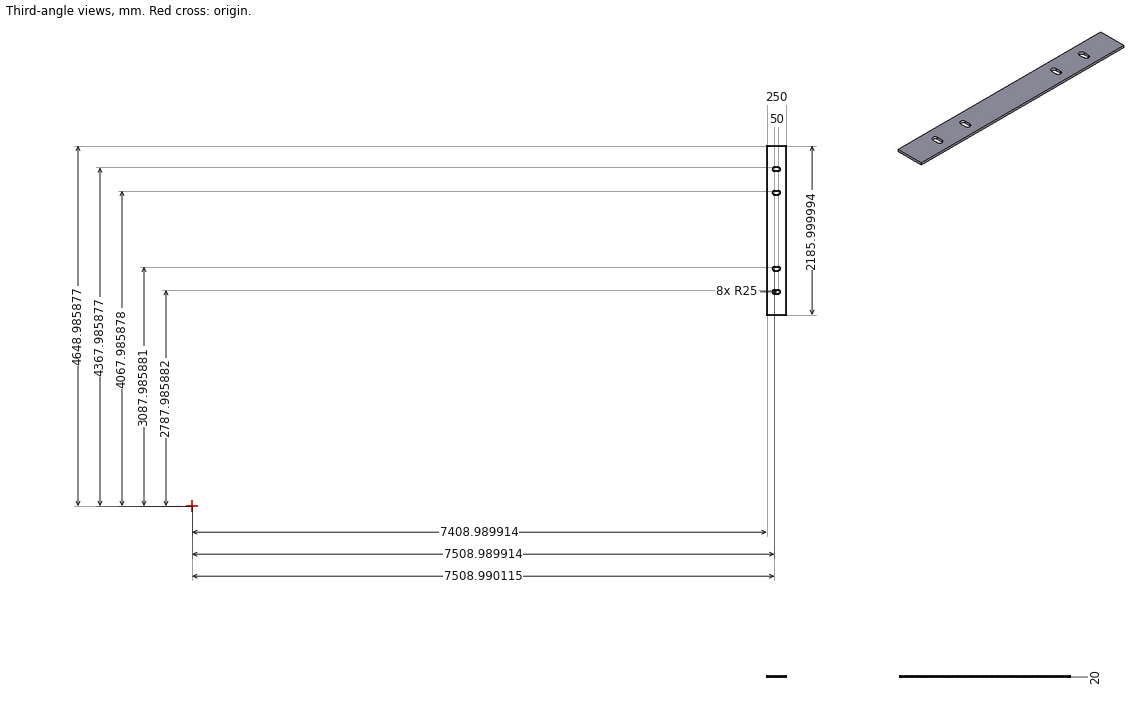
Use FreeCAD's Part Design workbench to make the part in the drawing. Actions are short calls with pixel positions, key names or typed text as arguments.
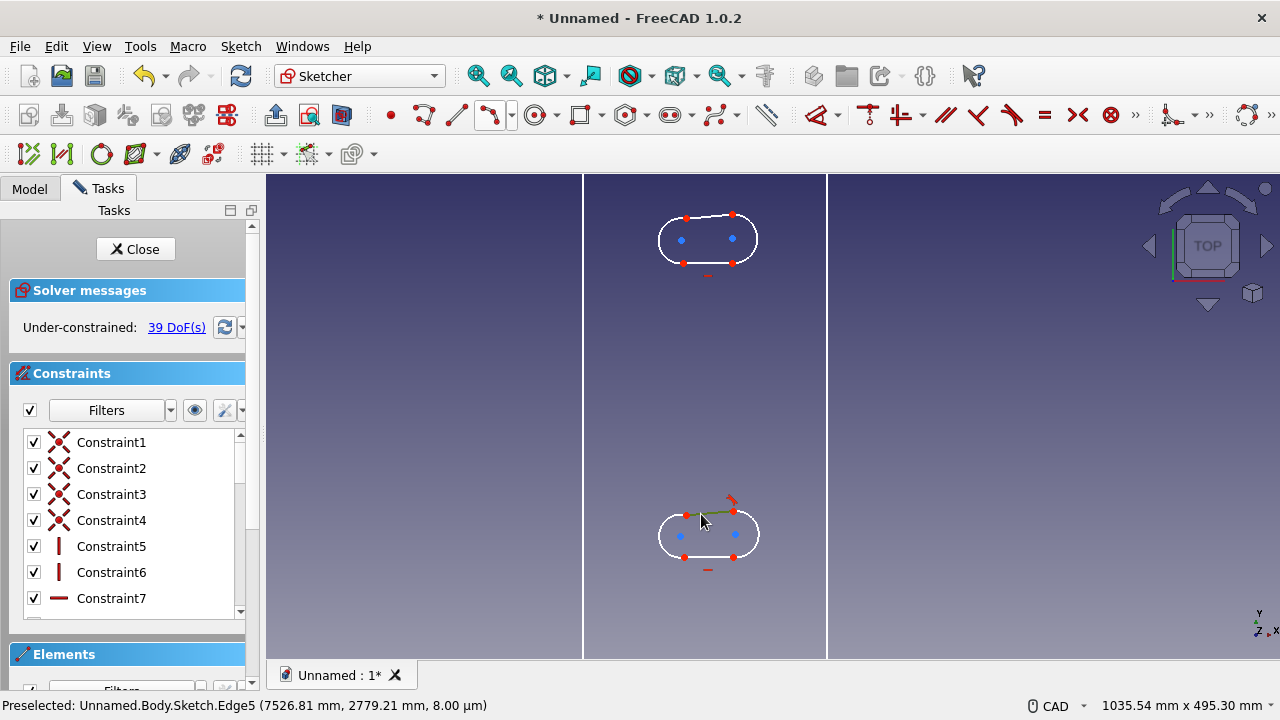
click(665, 521)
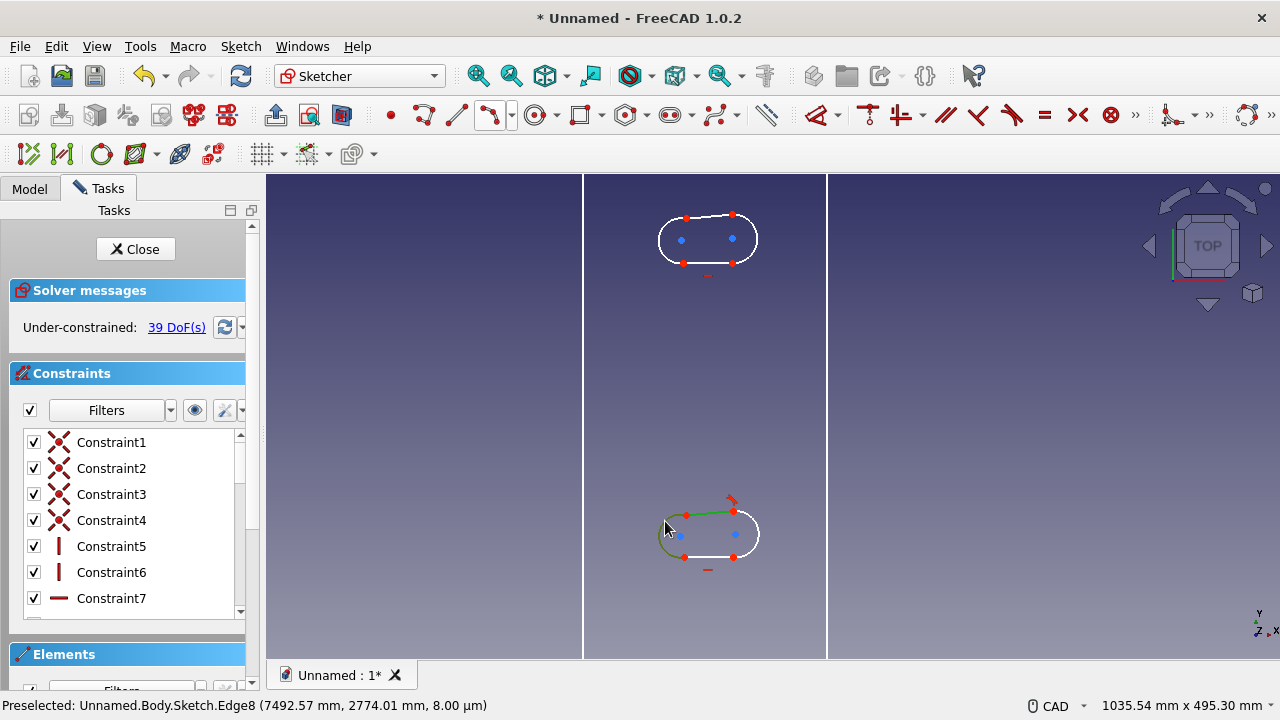
click(1012, 116)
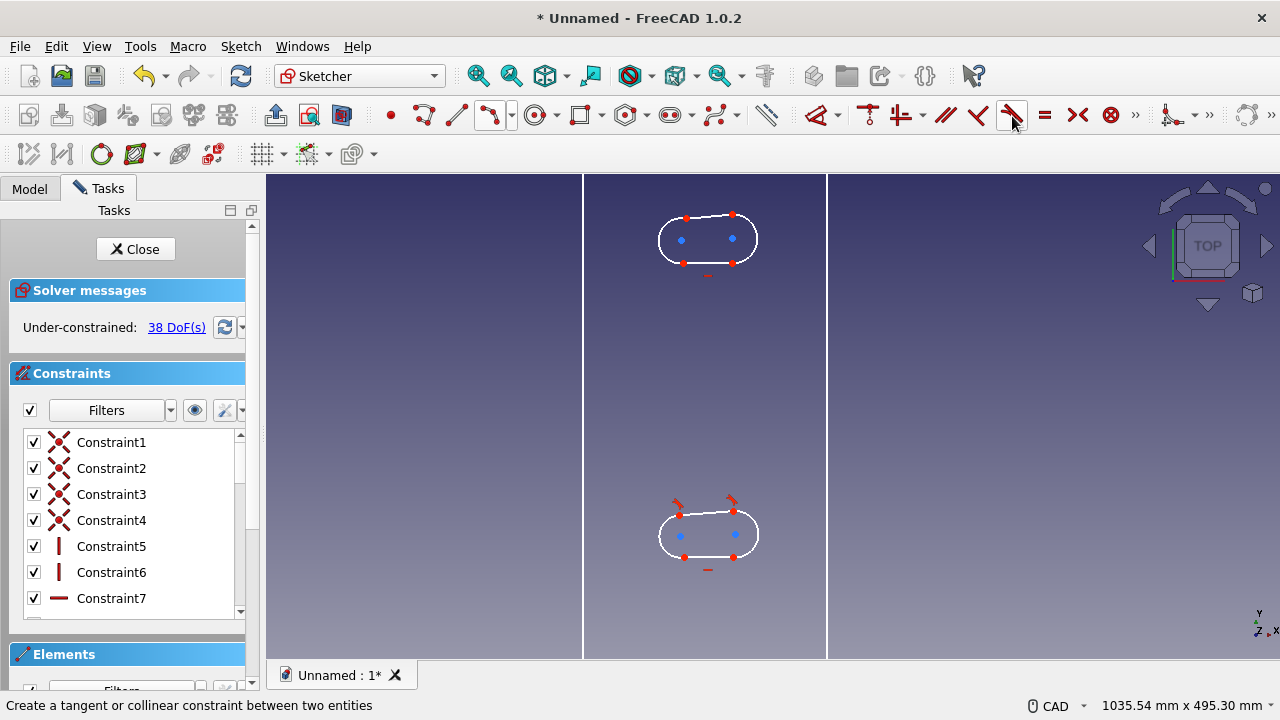
click(719, 557)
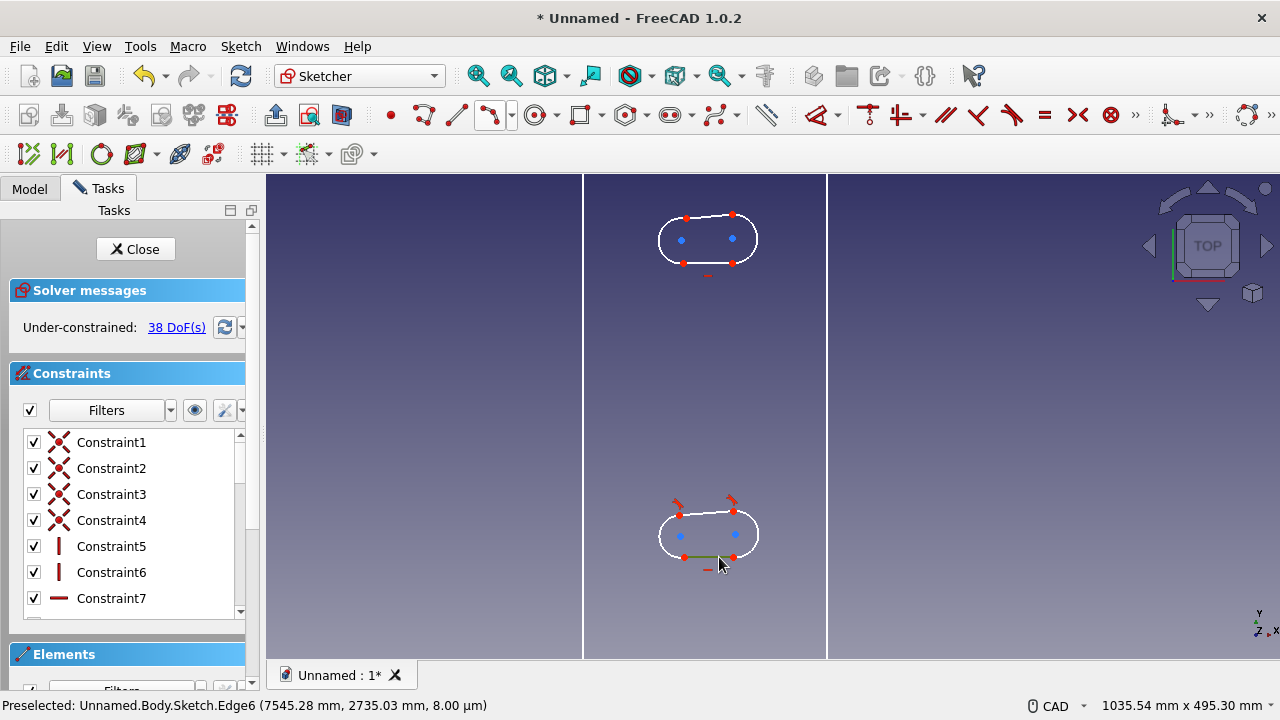
click(754, 548)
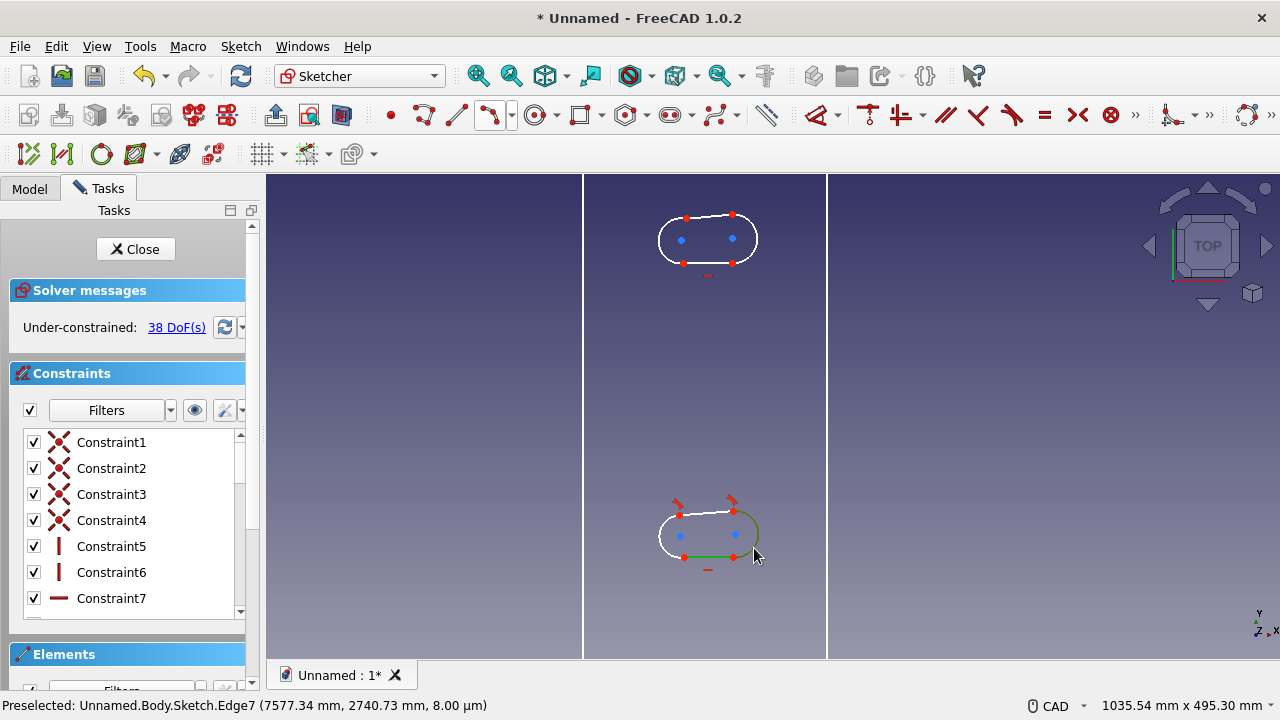
key(t)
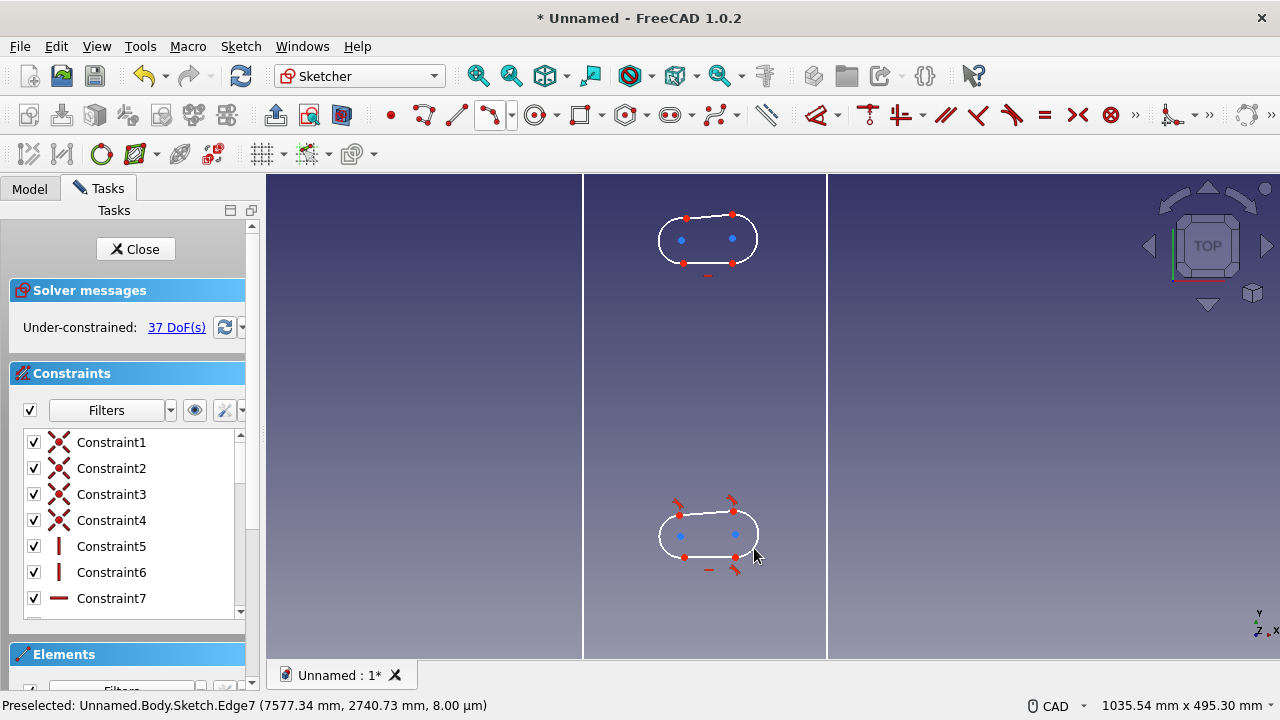
click(720, 557)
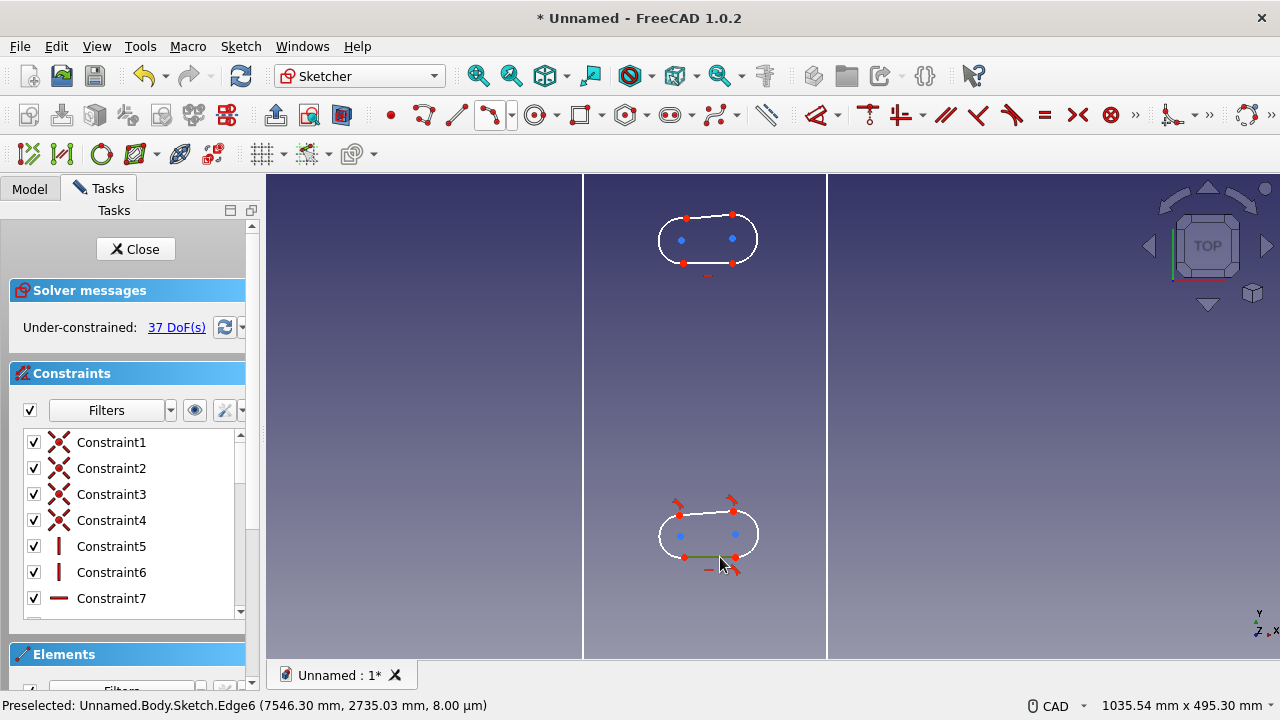
click(662, 526)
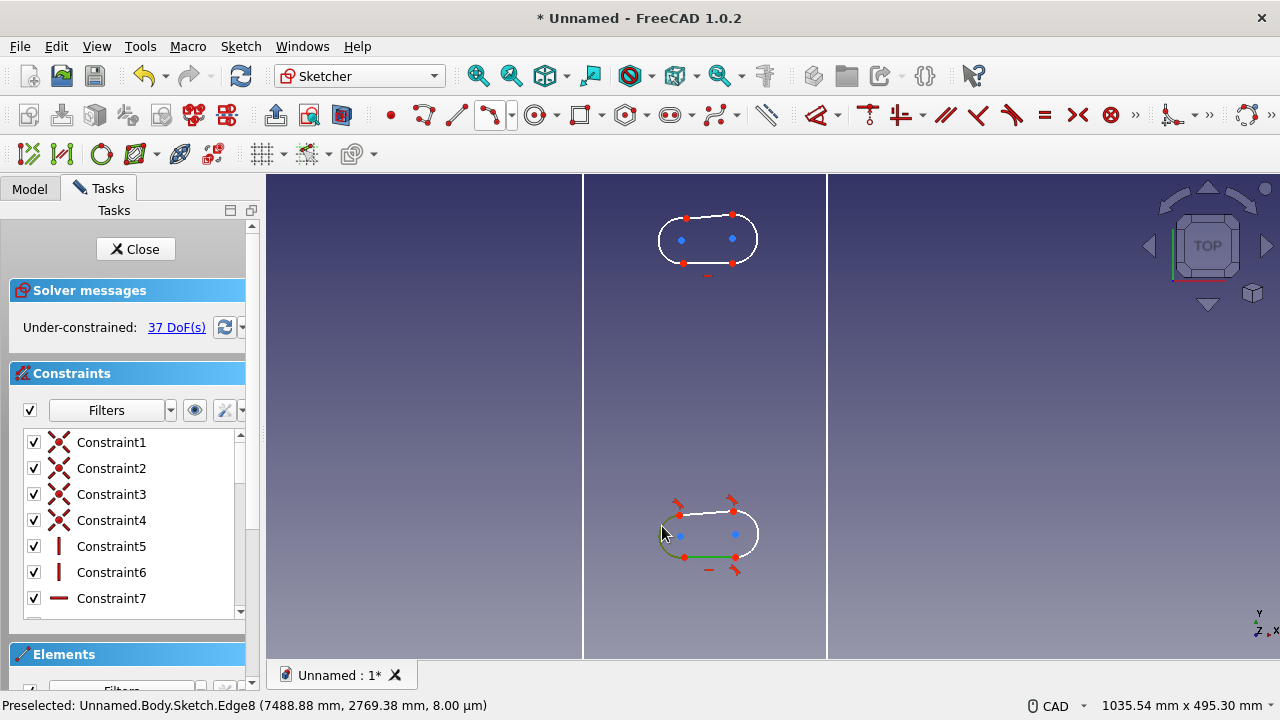
click(1012, 116)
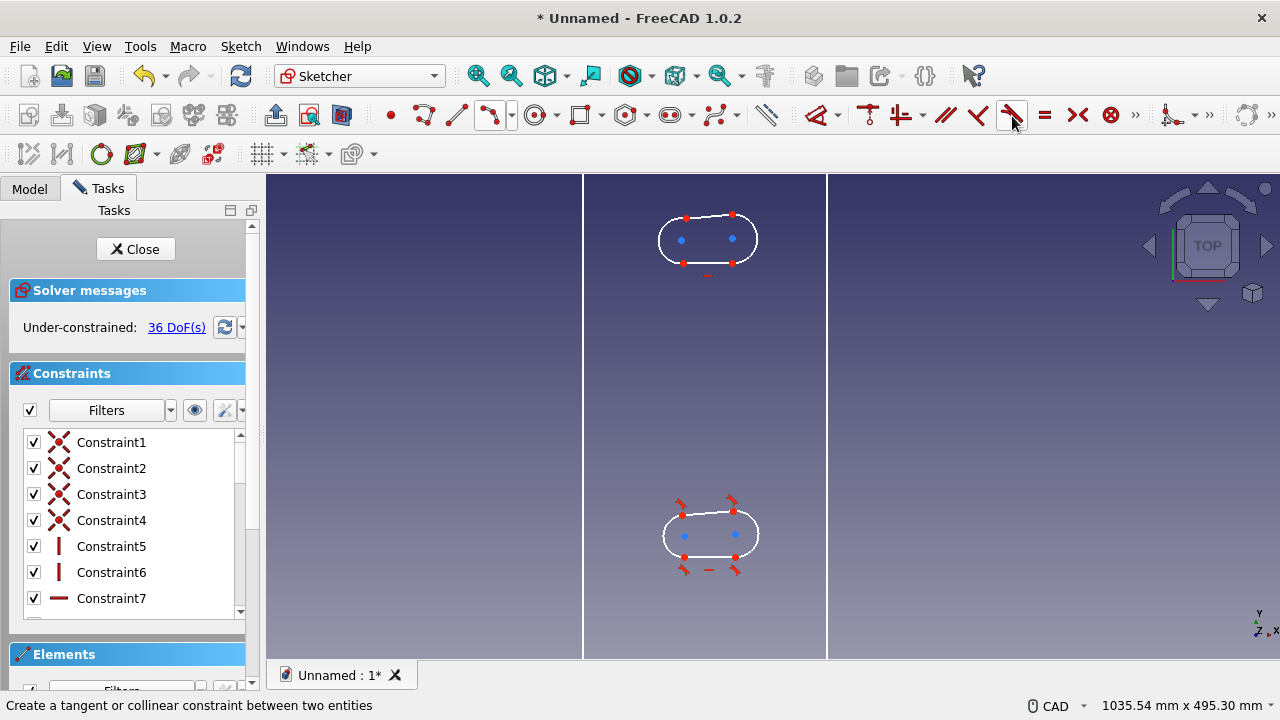
click(700, 218)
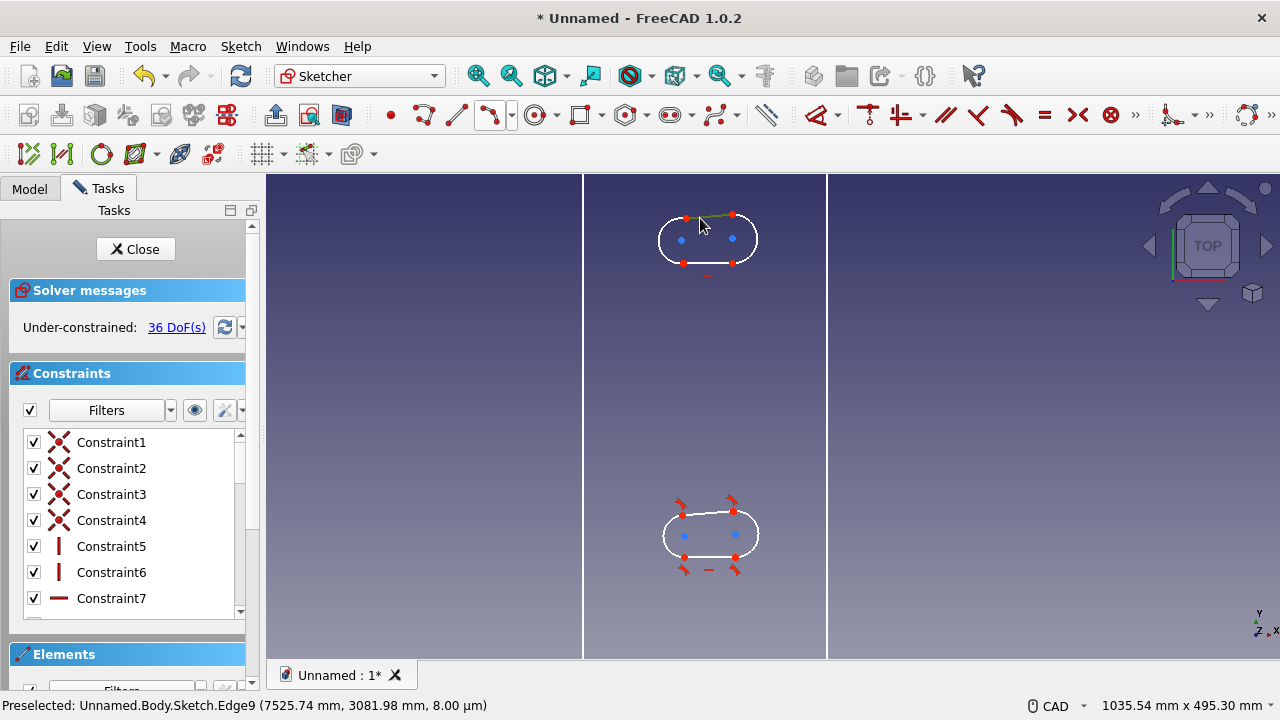
click(753, 253)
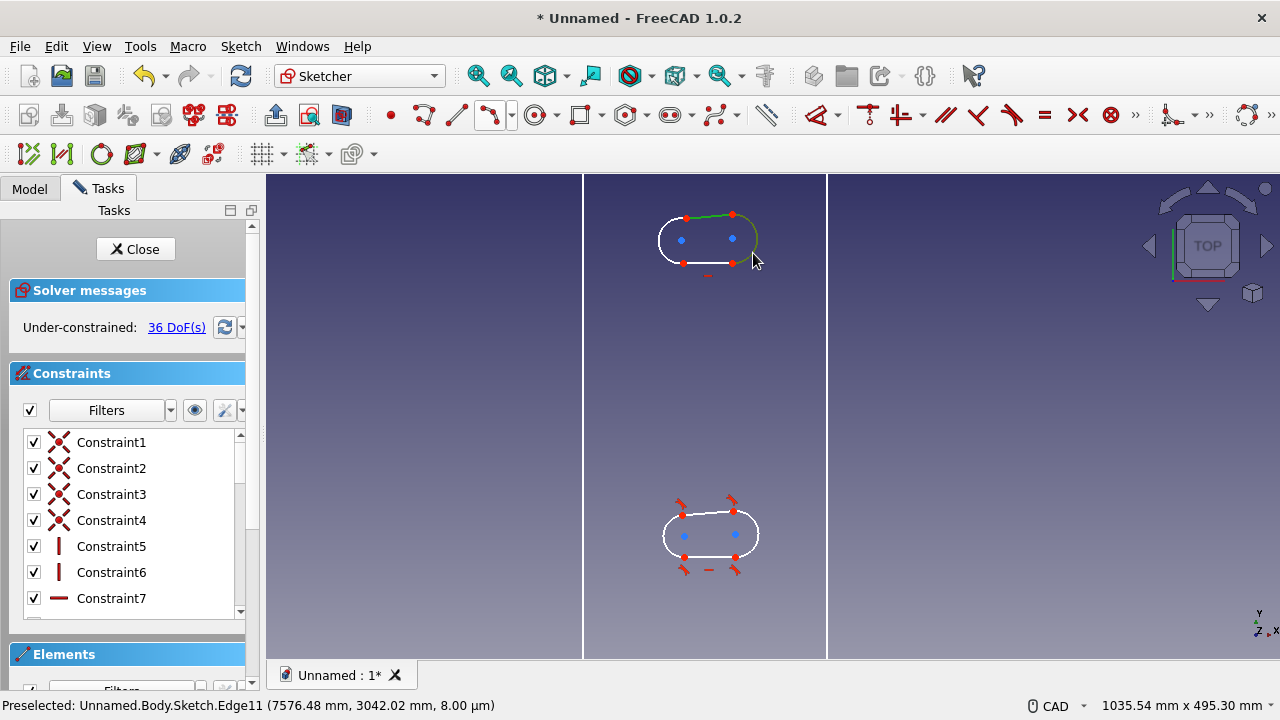
click(1012, 116)